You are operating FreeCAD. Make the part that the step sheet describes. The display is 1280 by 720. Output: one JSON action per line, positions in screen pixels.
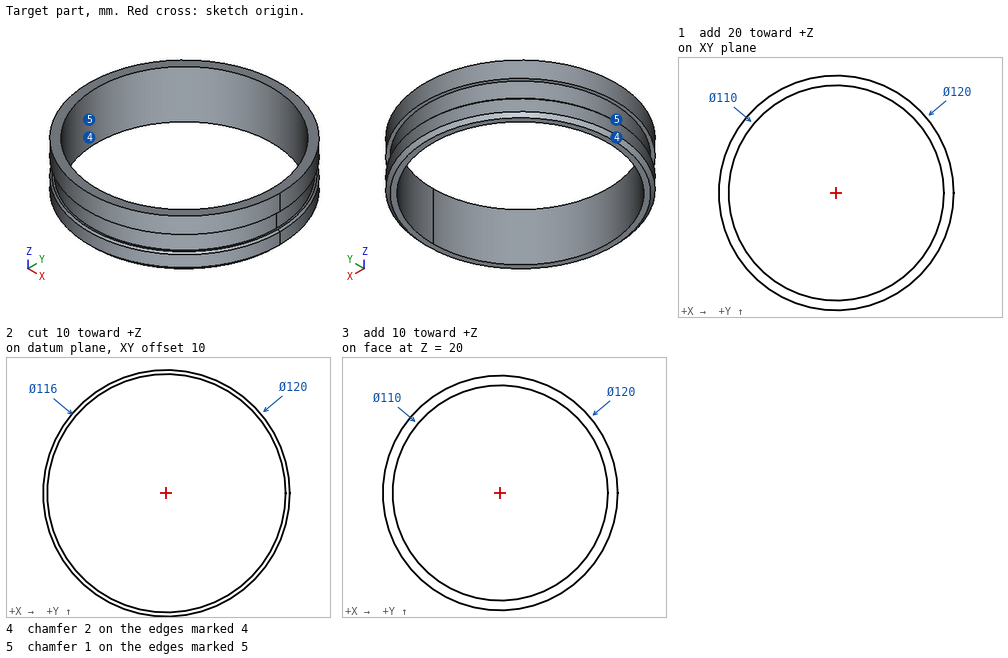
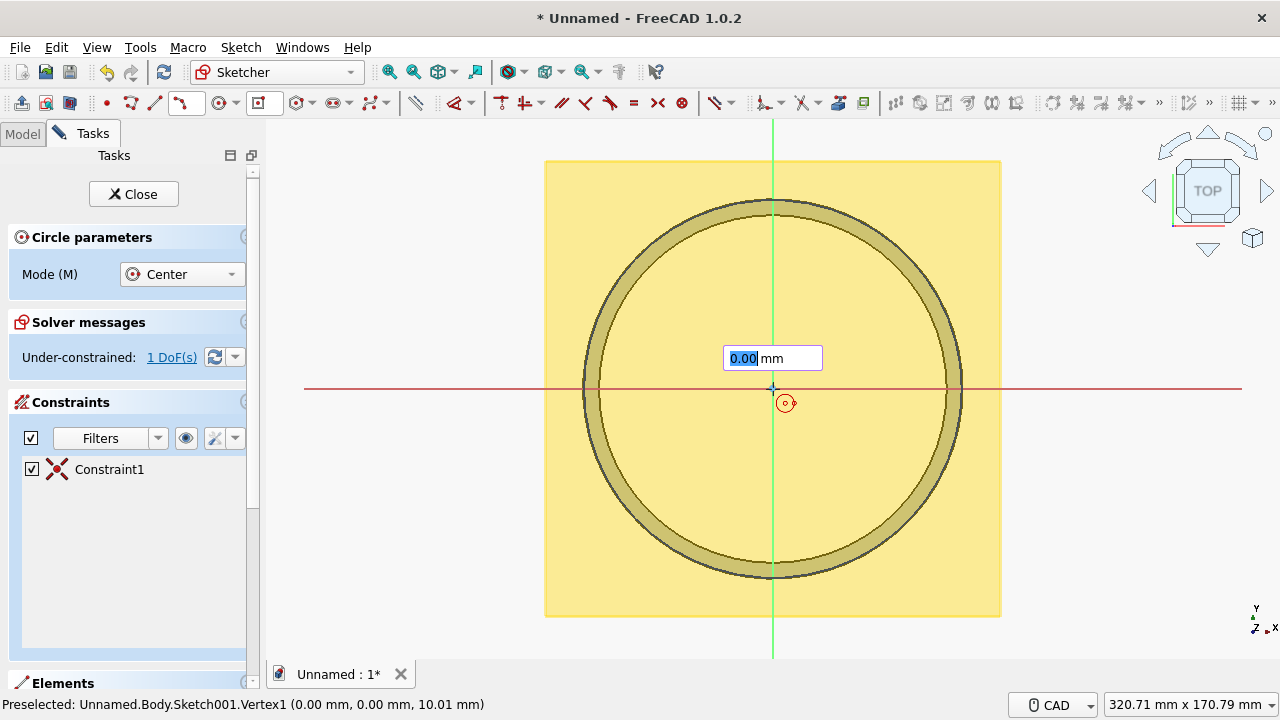
{"action": "scroll", "coordinate": [836, 217], "scroll_direction": "up", "scroll_amount": 5}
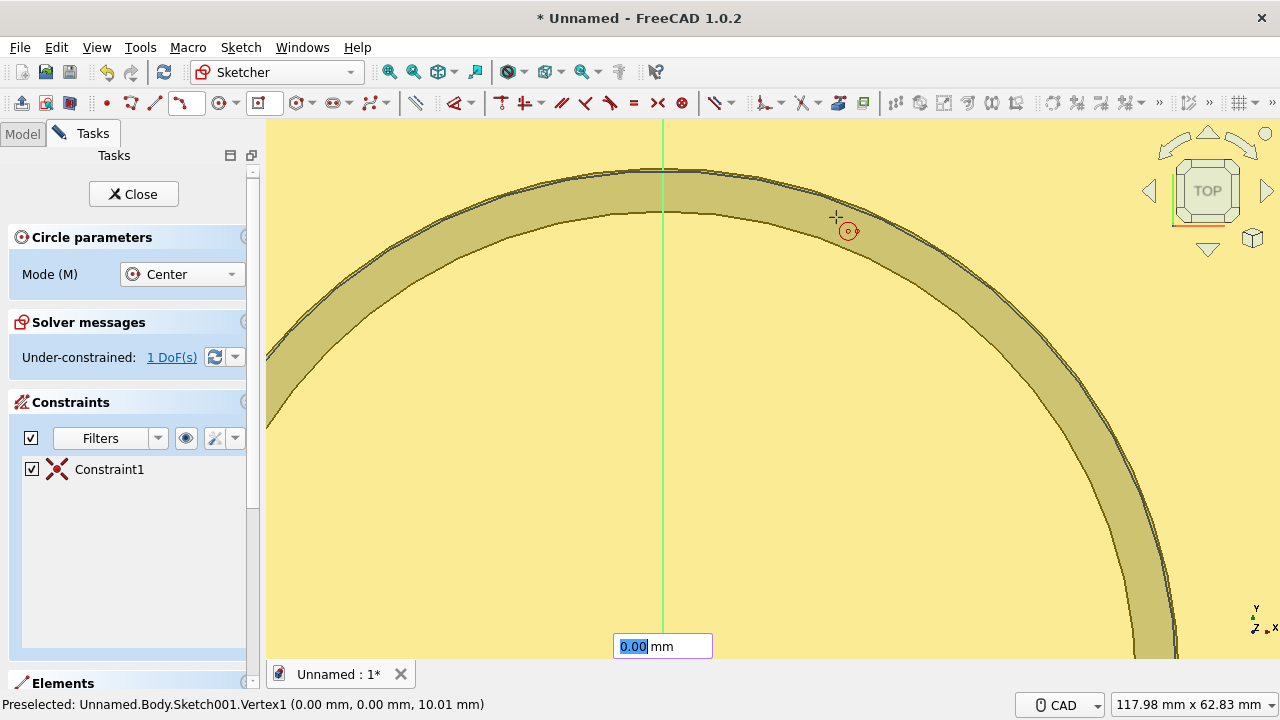
{"action": "left_click", "coordinate": [834, 216]}
{"action": "key", "text": "Escape"}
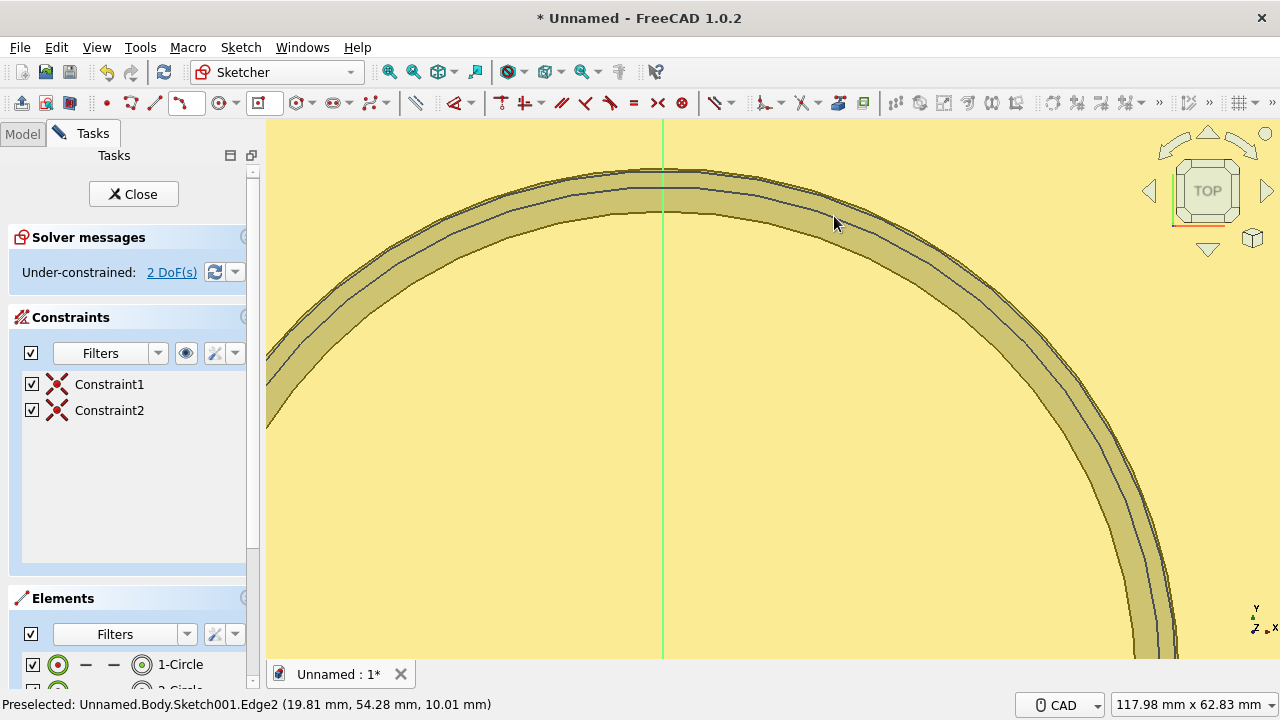
{"action": "left_click", "coordinate": [1025, 320]}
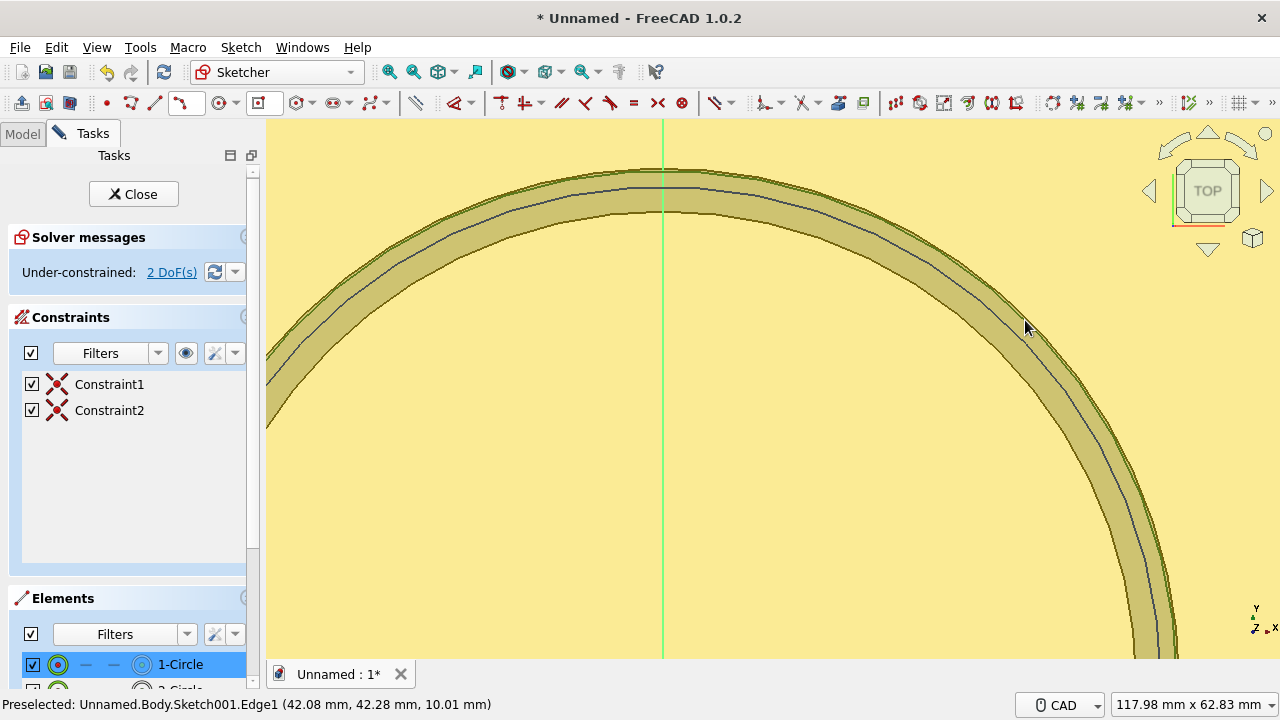
{"action": "key", "text": "k o"}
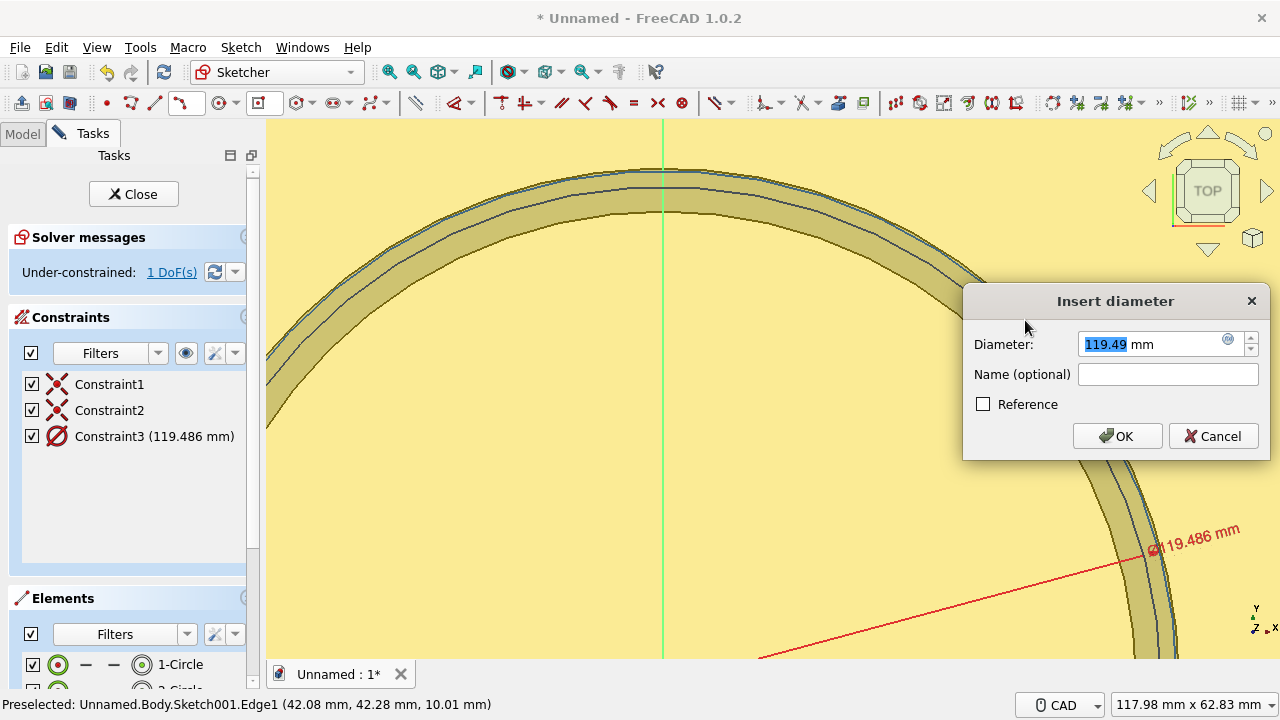
{"action": "type", "text": "120"}
{"action": "key", "text": "Return"}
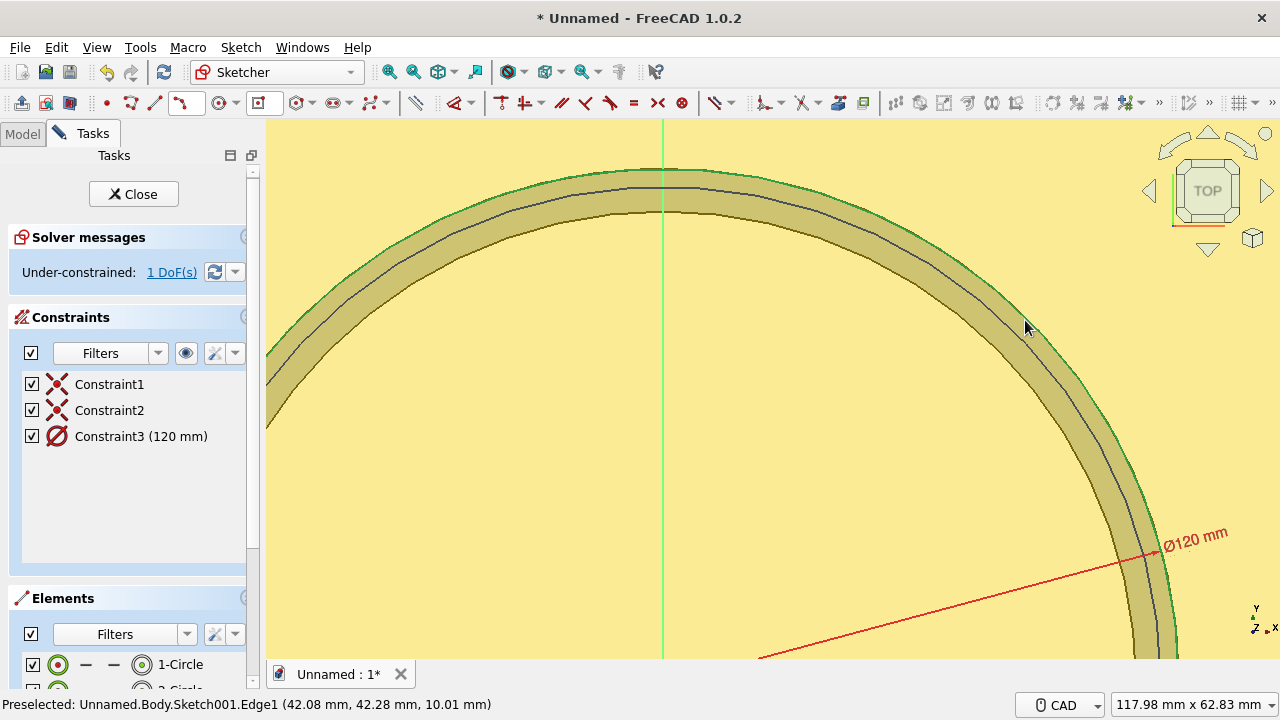
{"action": "left_click", "coordinate": [1014, 331]}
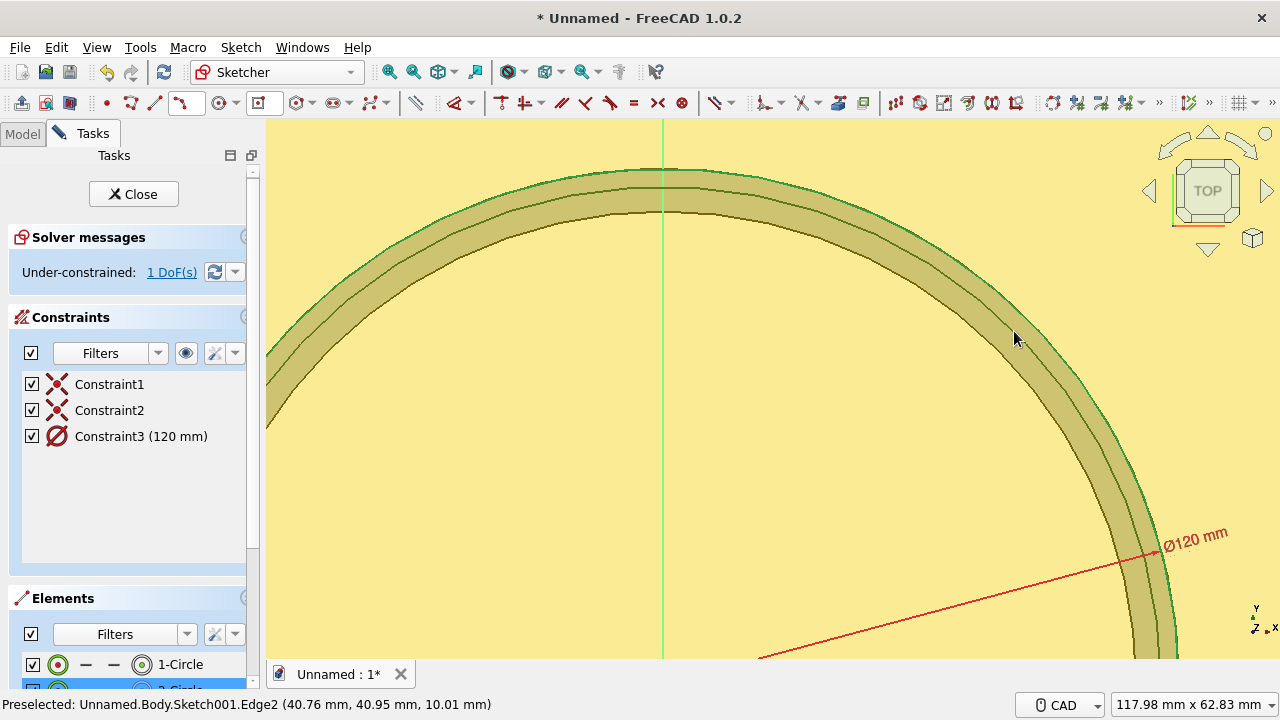
{"action": "key", "text": "k o"}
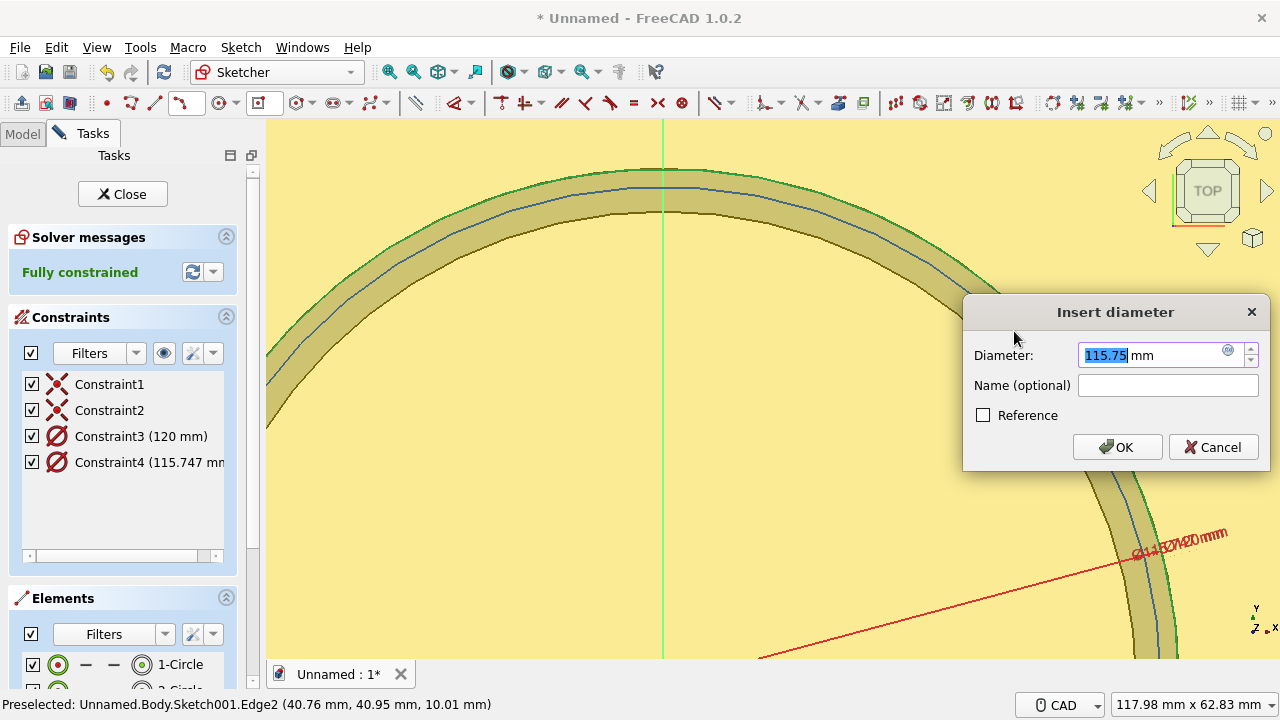
{"action": "type", "text": "116"}
{"action": "key", "text": "Return"}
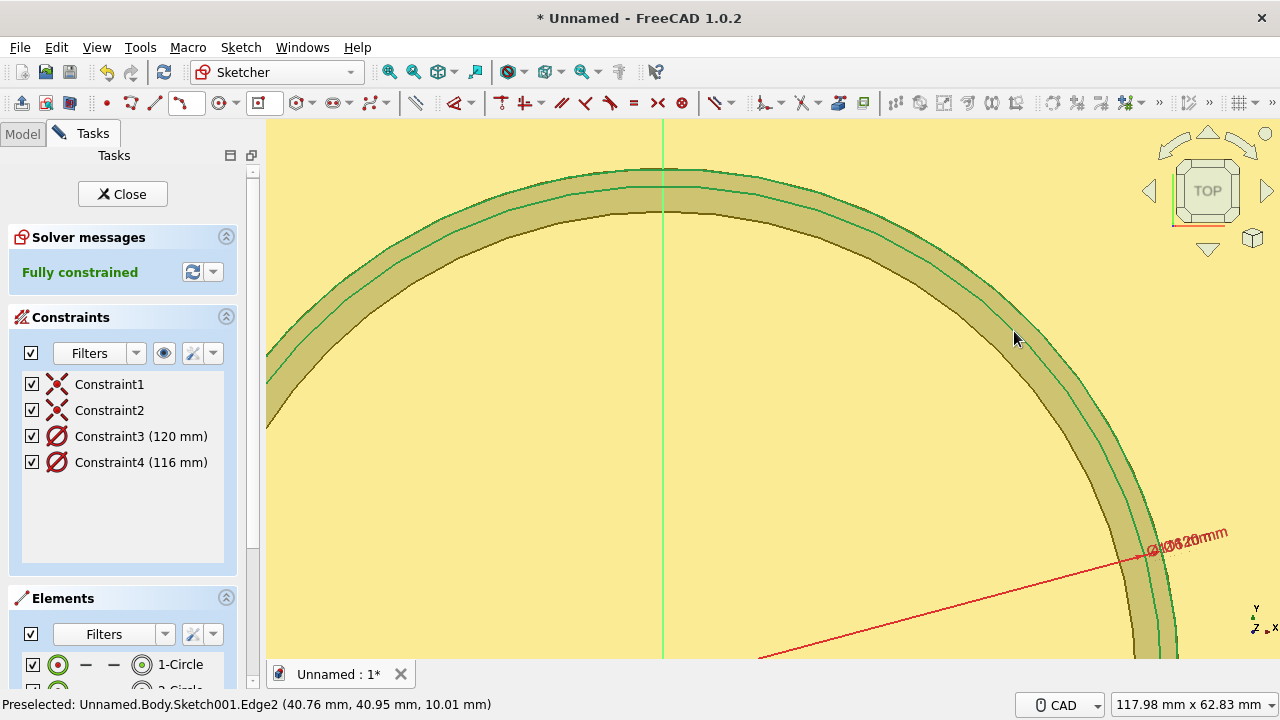
{"action": "left_click", "coordinate": [123, 194]}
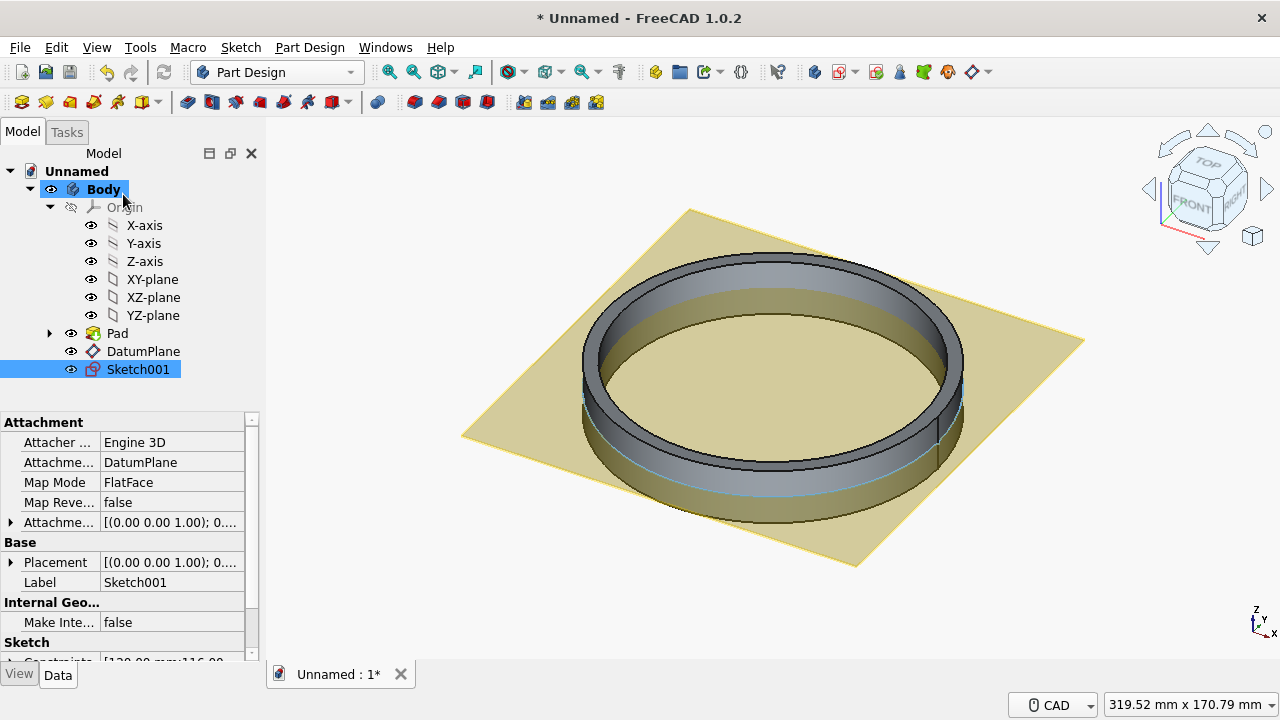
{"action": "left_click", "coordinate": [188, 102]}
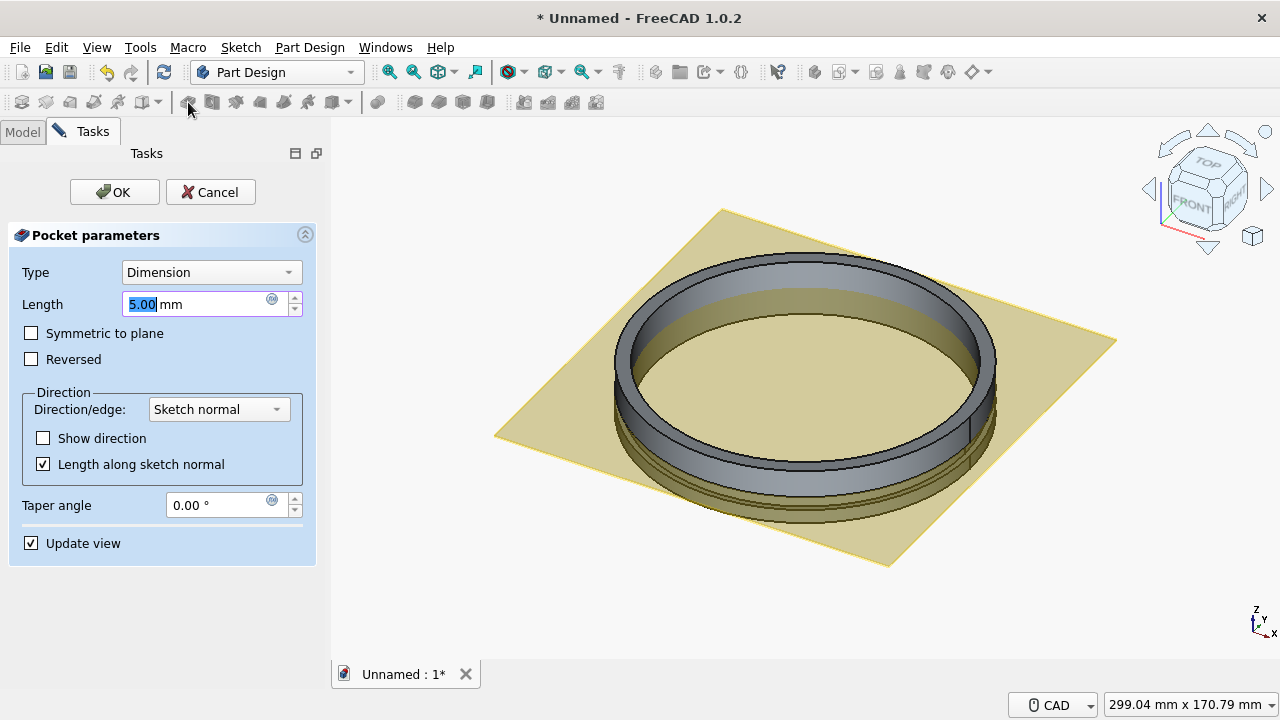
{"action": "type", "text": "10"}
{"action": "key", "text": "Tab"}